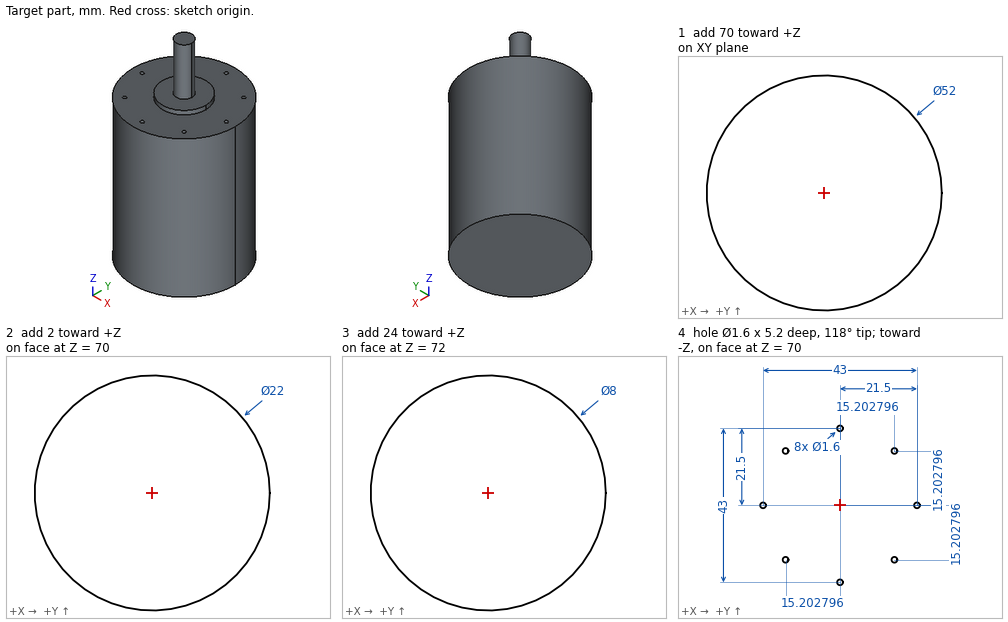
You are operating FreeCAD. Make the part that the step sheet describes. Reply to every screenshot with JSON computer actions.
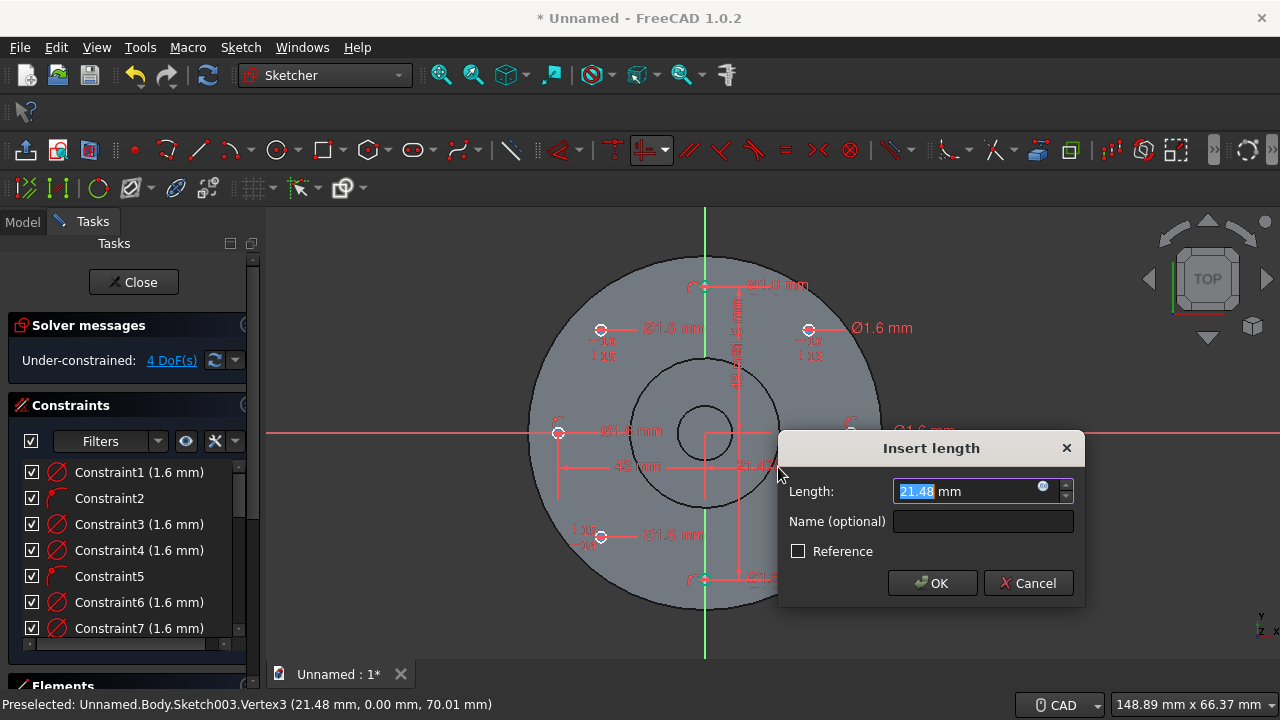
{"action": "type", "text": "21.5"}
{"action": "key", "text": "Return"}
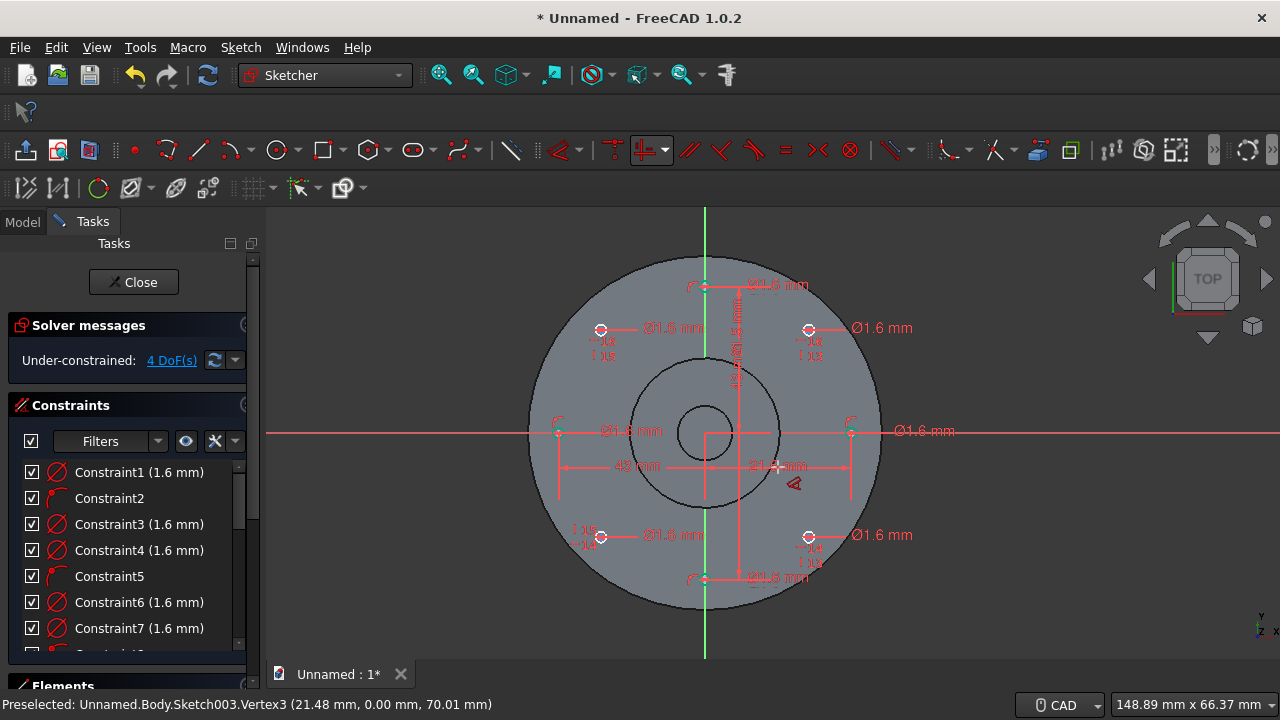
{"action": "left_click", "coordinate": [809, 330]}
{"action": "left_click", "coordinate": [757, 296]}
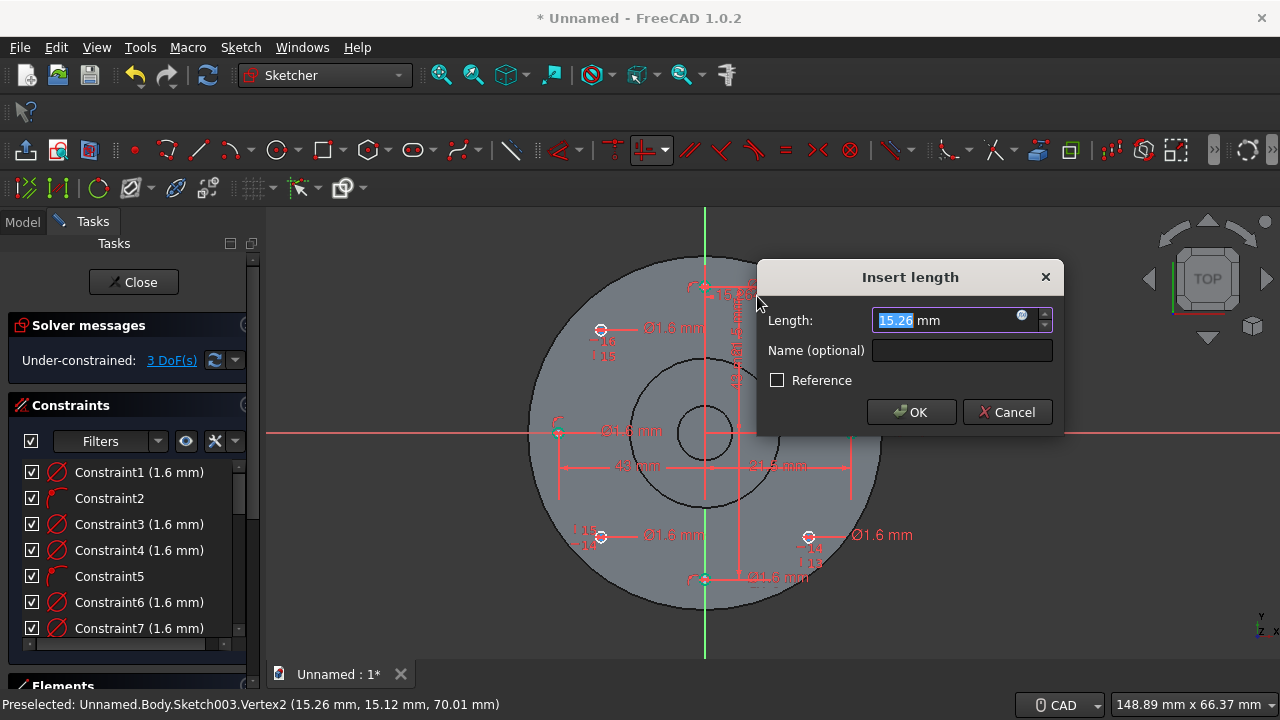
{"action": "type", "text": "15.202796"}
{"action": "key", "text": "Return"}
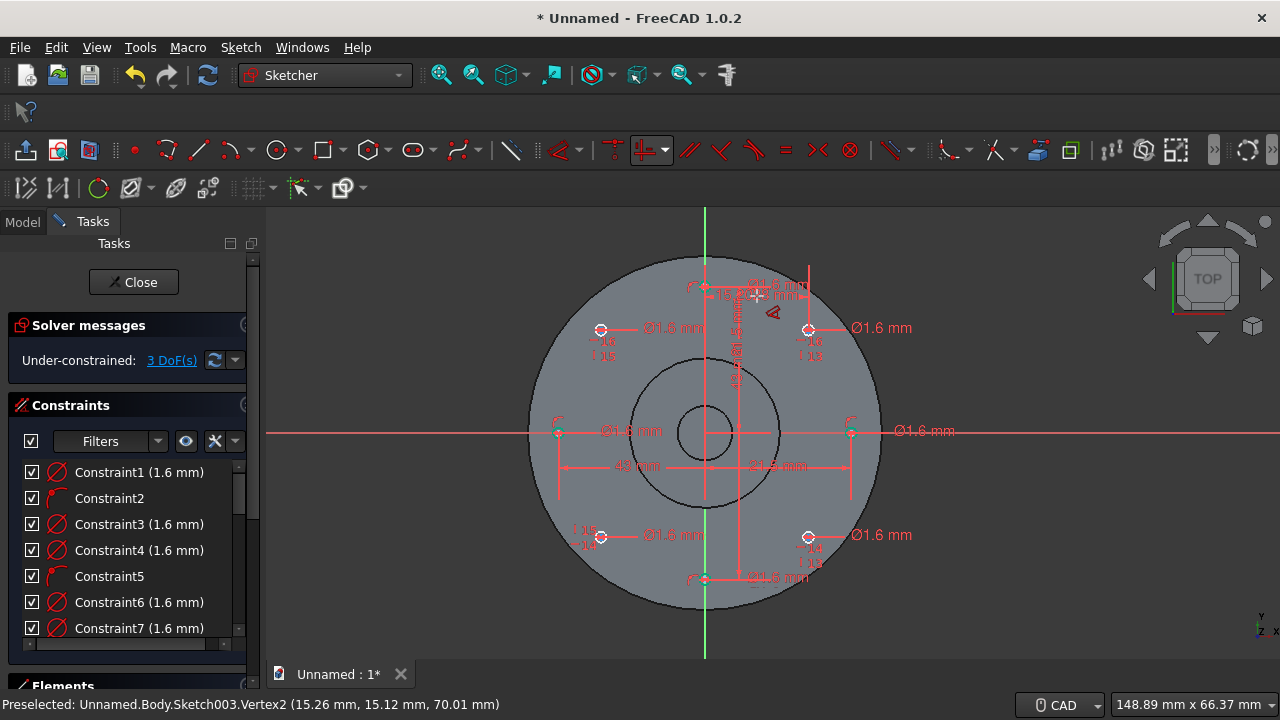
{"action": "left_click", "coordinate": [809, 330]}
{"action": "left_click", "coordinate": [843, 382]}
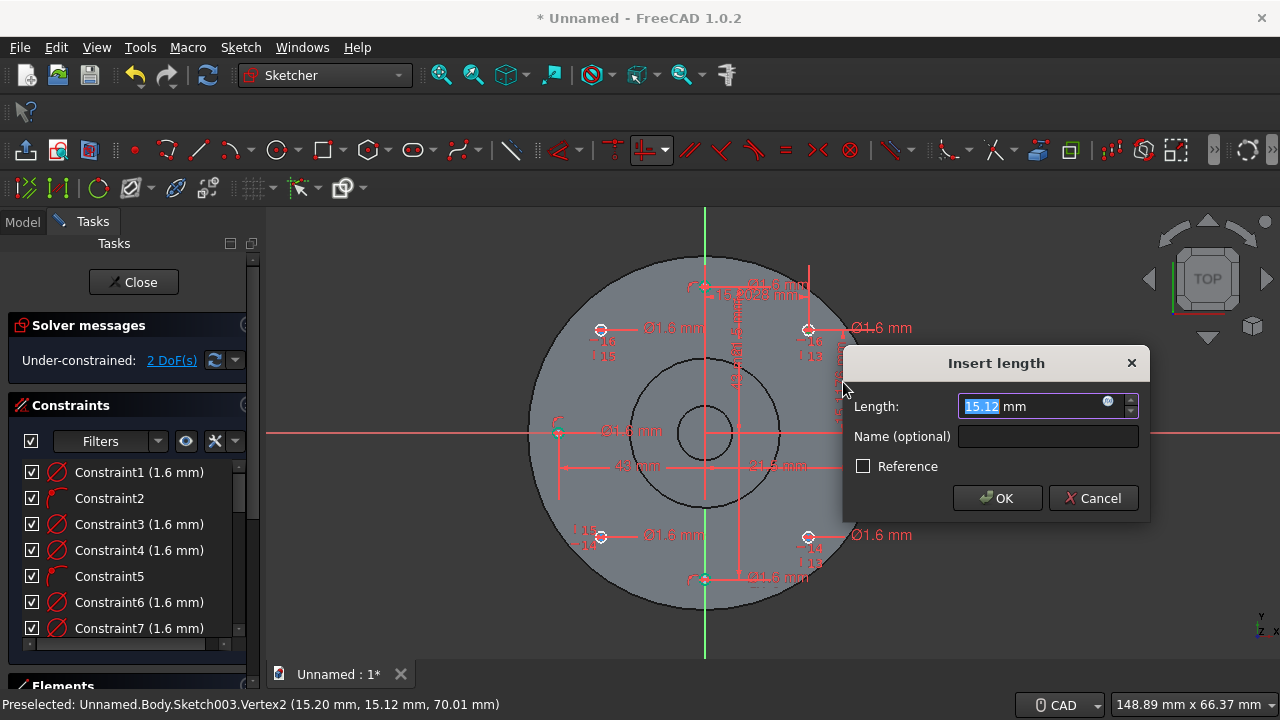
{"action": "type", "text": "15.202796"}
{"action": "key", "text": "Return"}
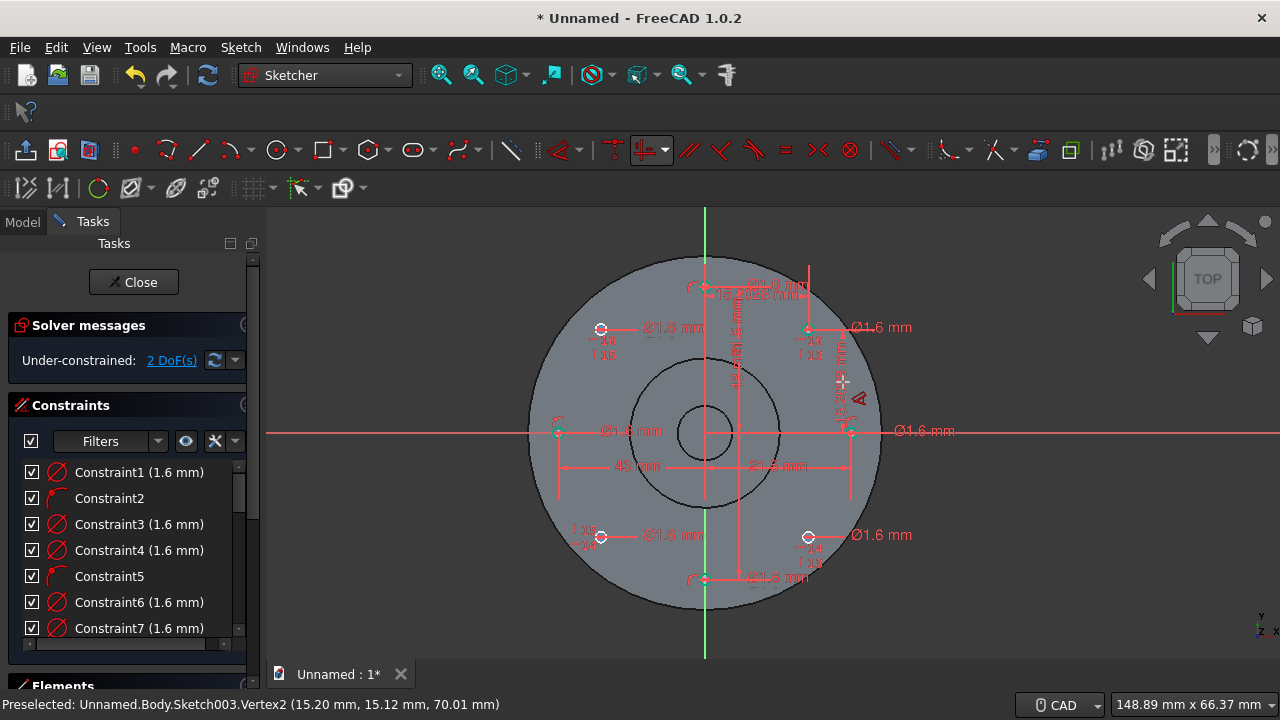
{"action": "left_click", "coordinate": [809, 537]}
{"action": "left_click", "coordinate": [843, 509]}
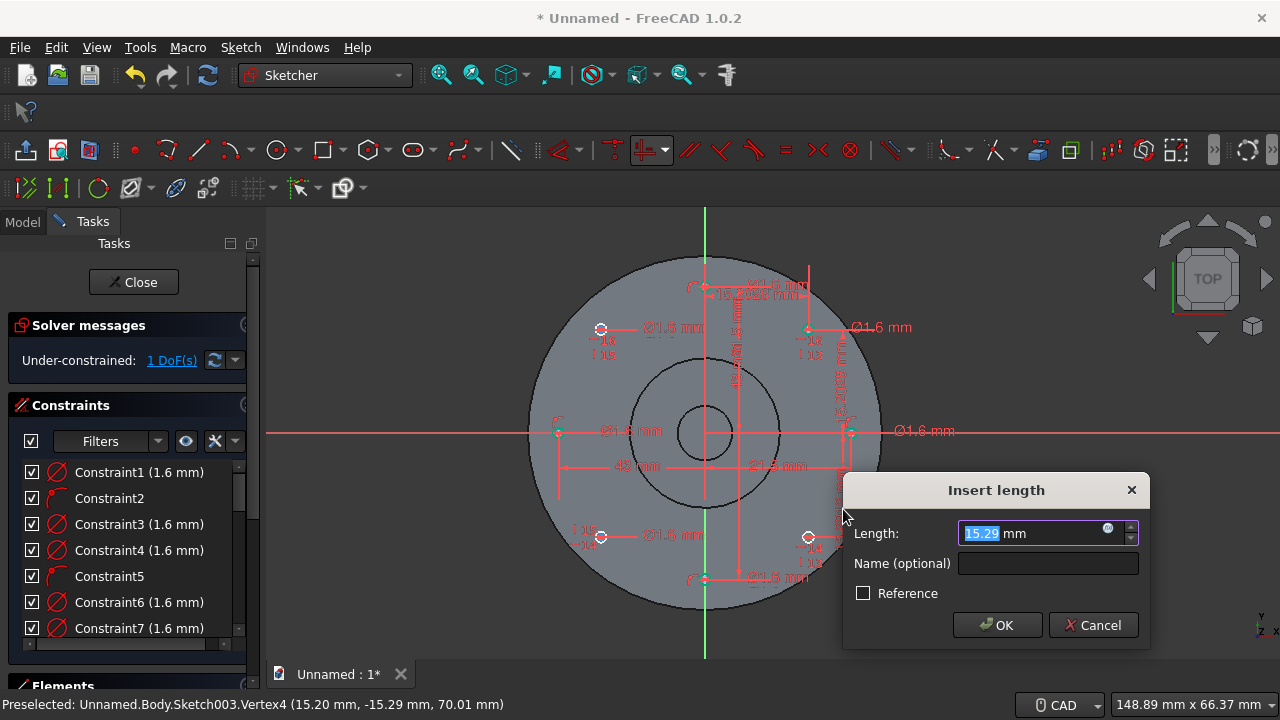
{"action": "type", "text": "15.202796"}
{"action": "key", "text": "Return"}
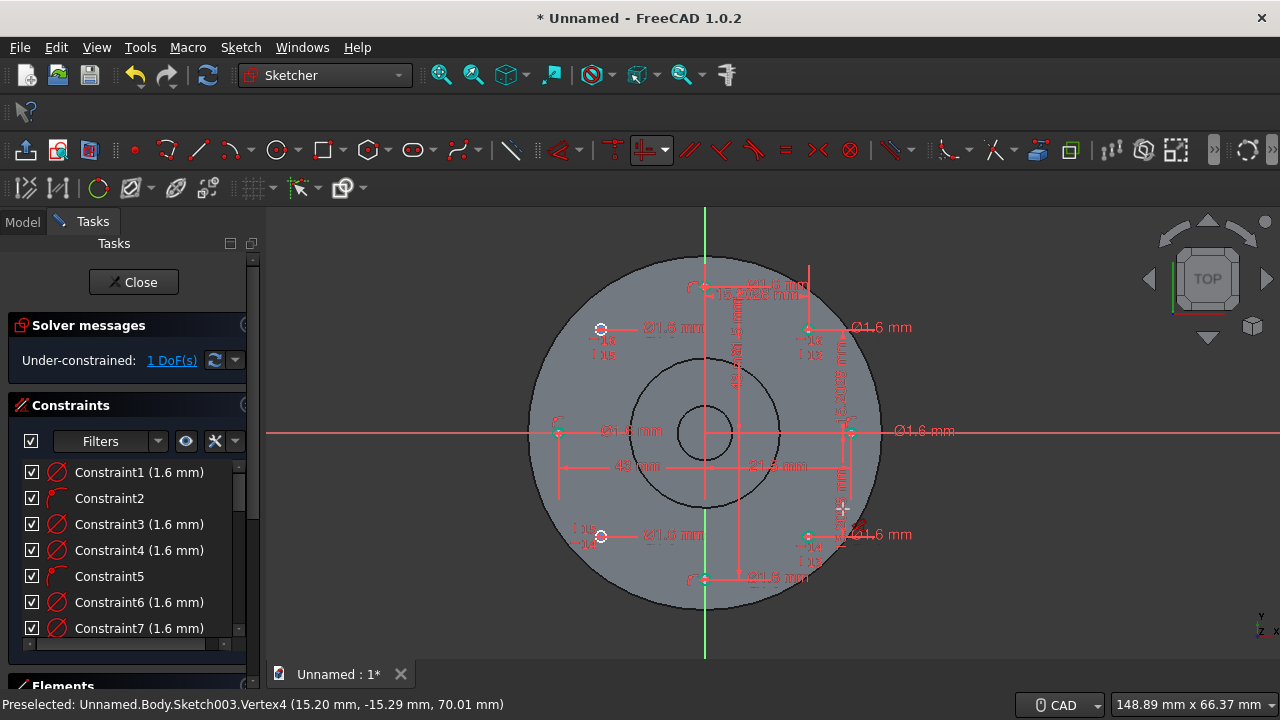
{"action": "left_click", "coordinate": [601, 537]}
{"action": "left_click", "coordinate": [653, 571]}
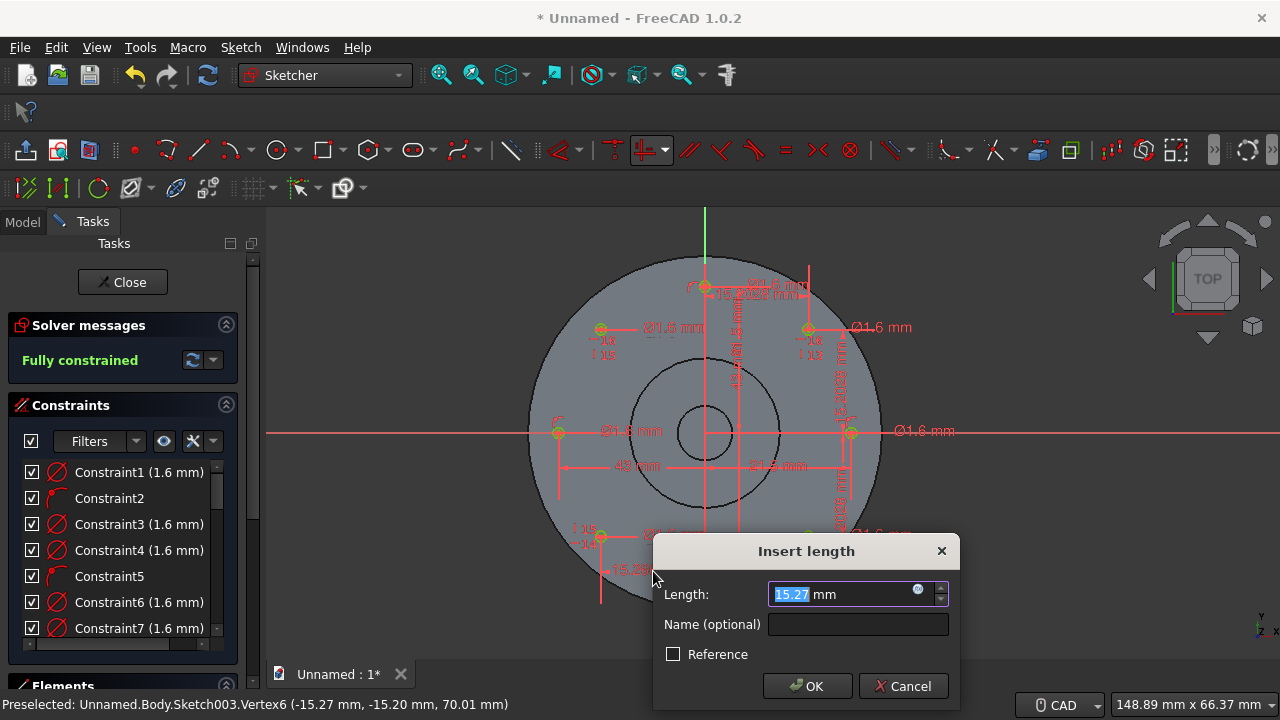
{"action": "type", "text": "15.202796"}
{"action": "key", "text": "Return"}
{"action": "key", "text": "Escape"}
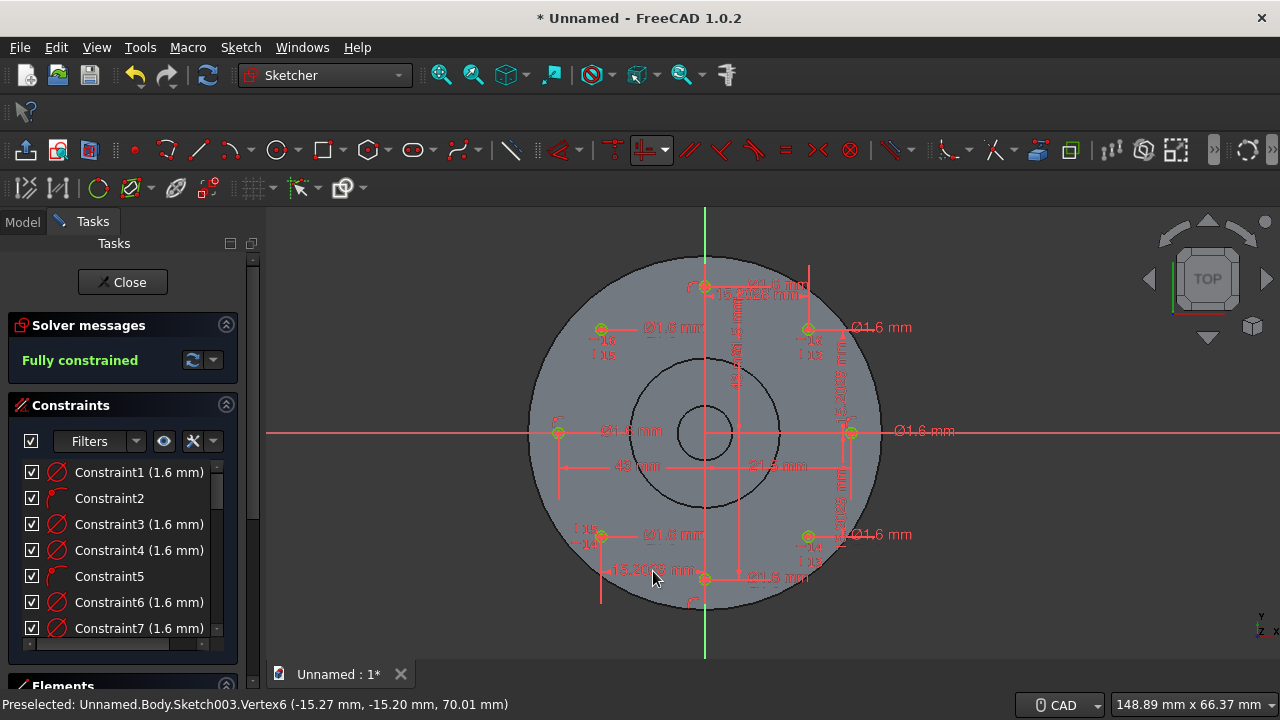
{"action": "left_click", "coordinate": [123, 282]}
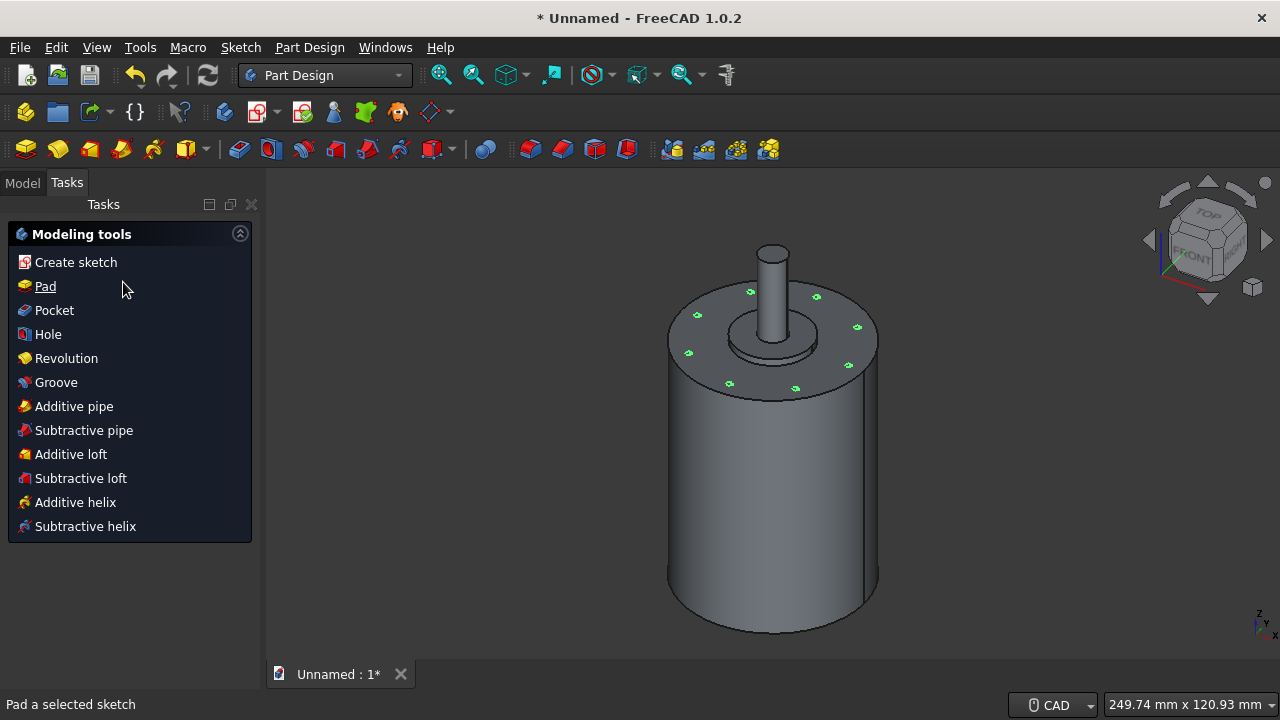
{"action": "left_click", "coordinate": [272, 150]}